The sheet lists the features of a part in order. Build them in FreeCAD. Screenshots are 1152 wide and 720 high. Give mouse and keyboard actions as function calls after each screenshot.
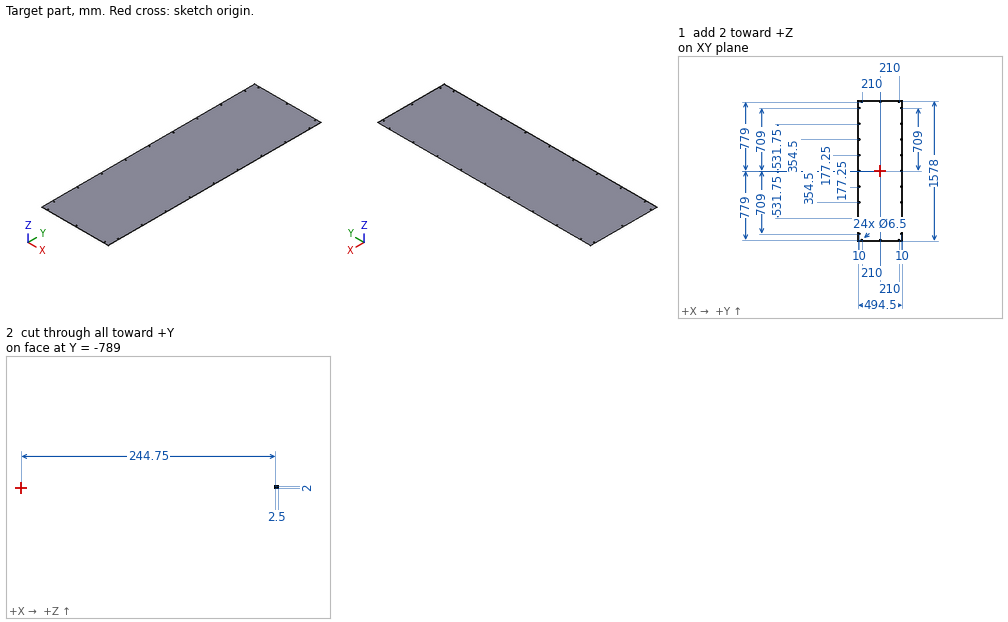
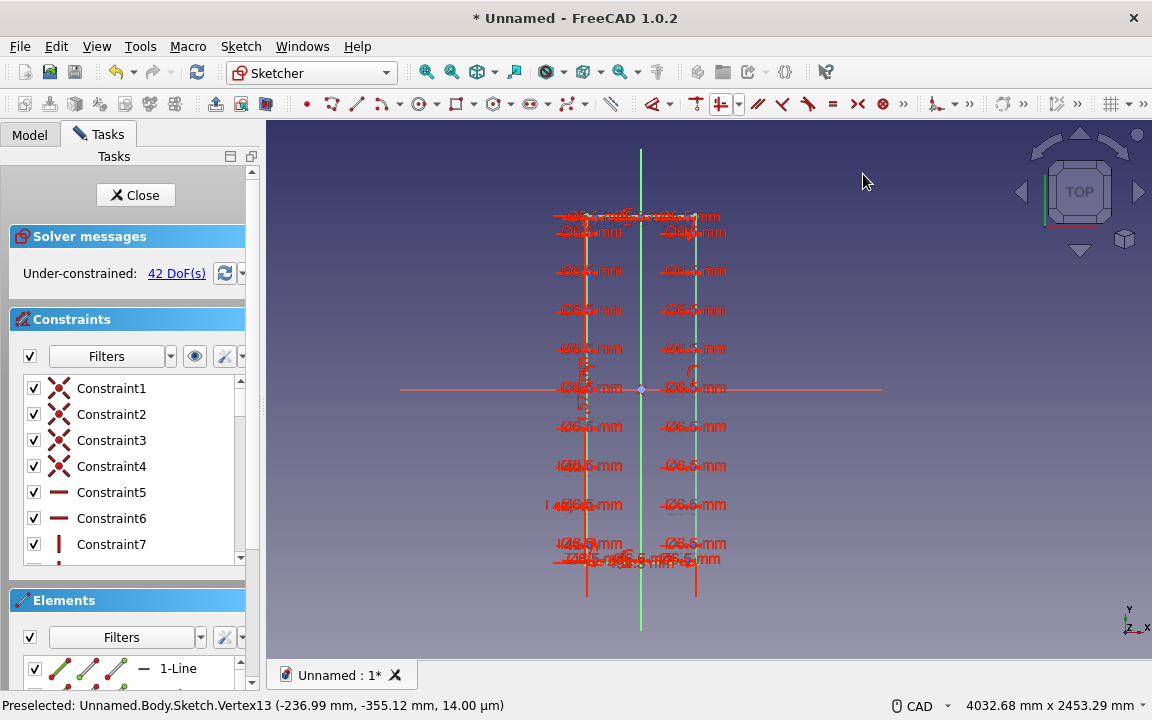
click(589, 468)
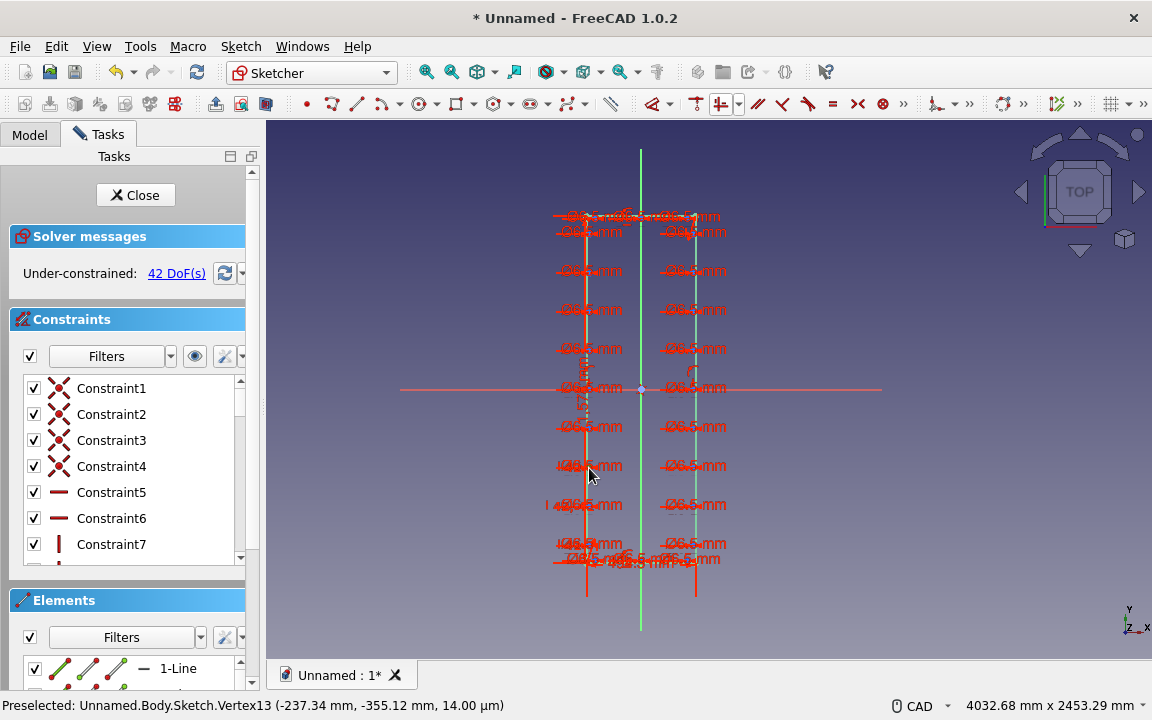
click(589, 429)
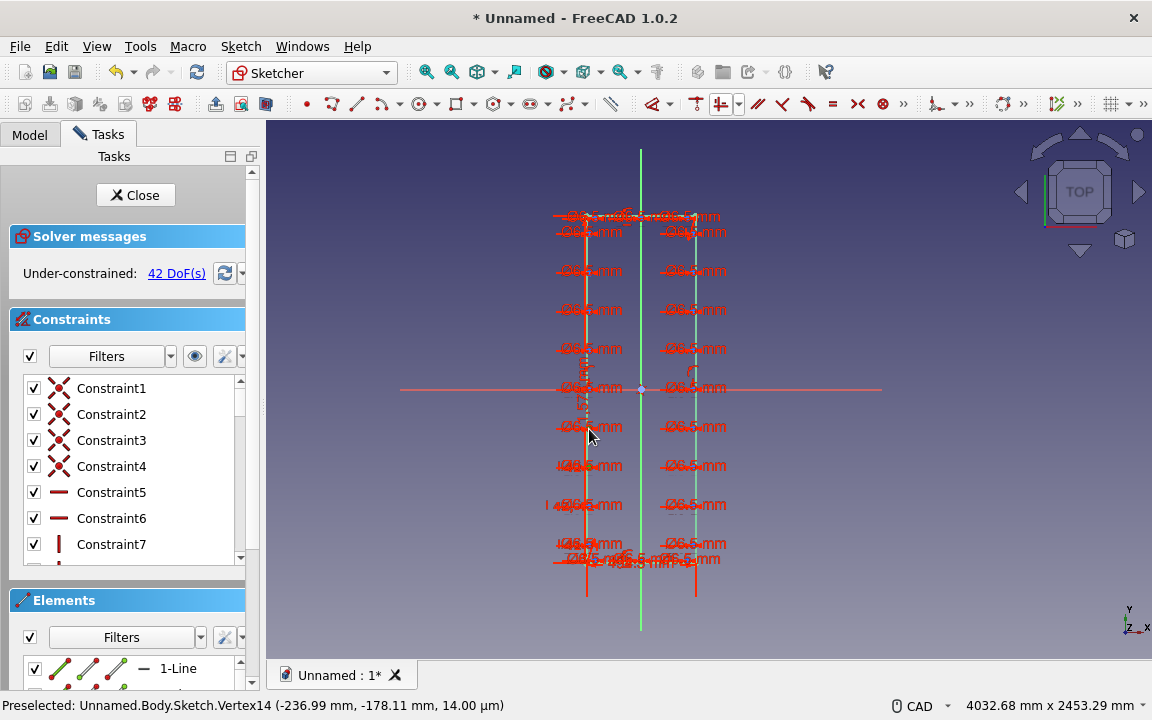
key(v)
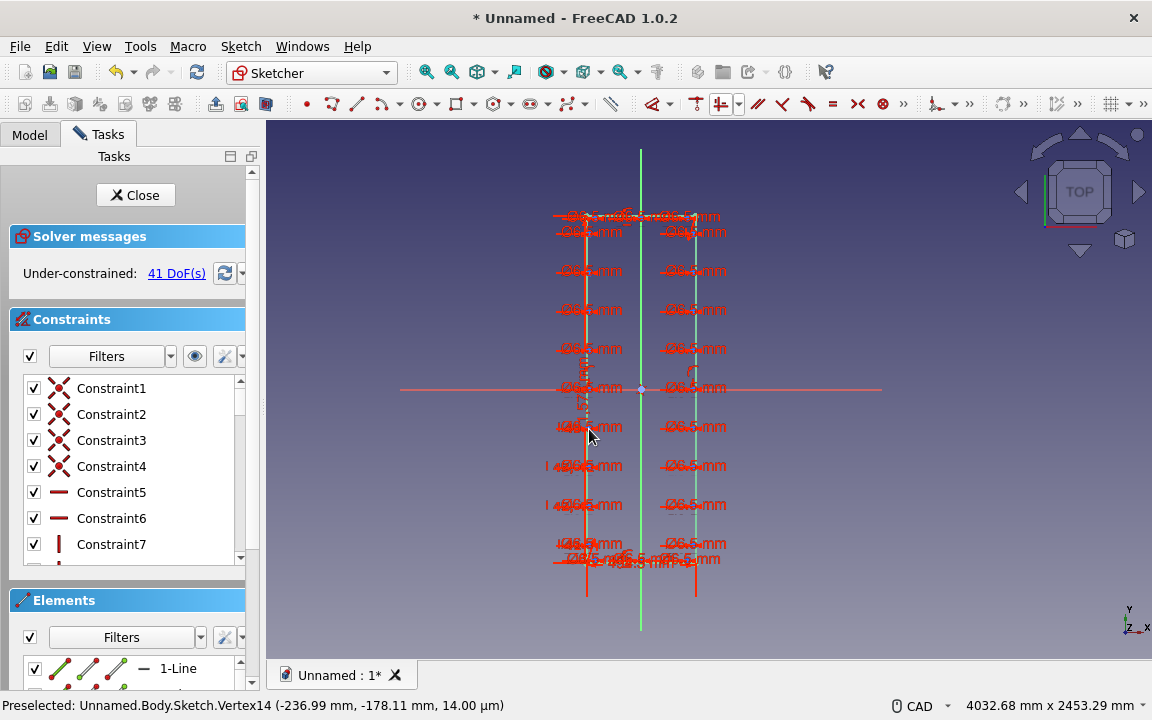
scroll(595, 561, up, 2)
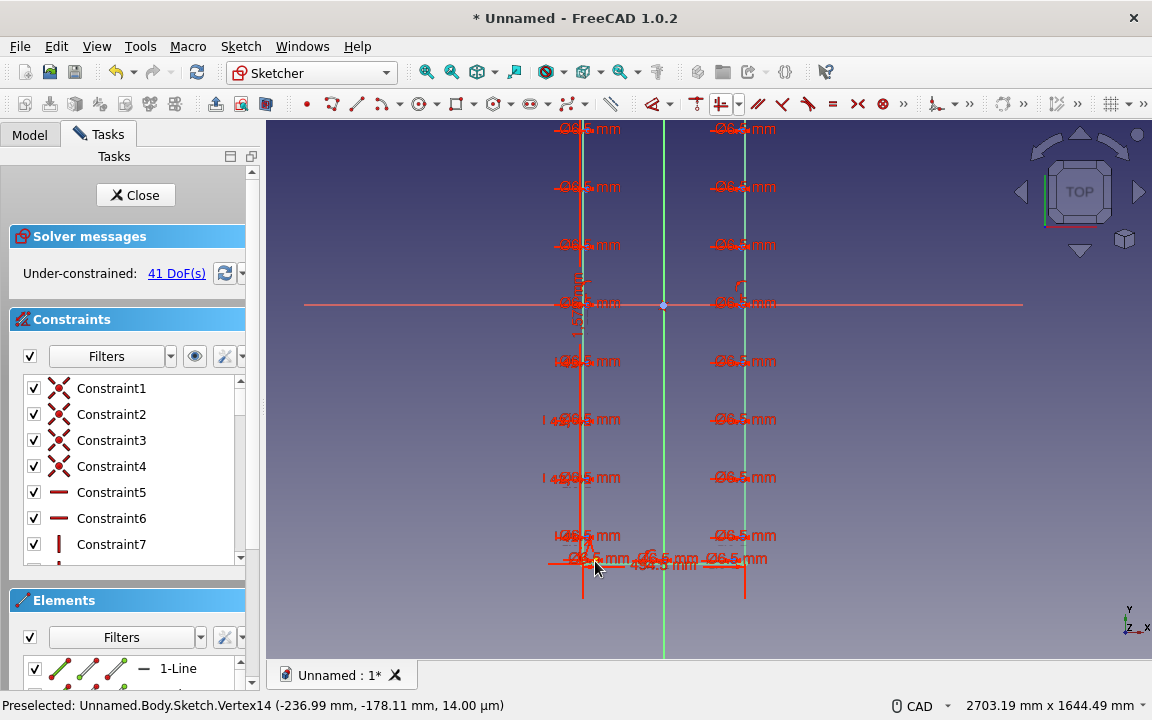
click(595, 560)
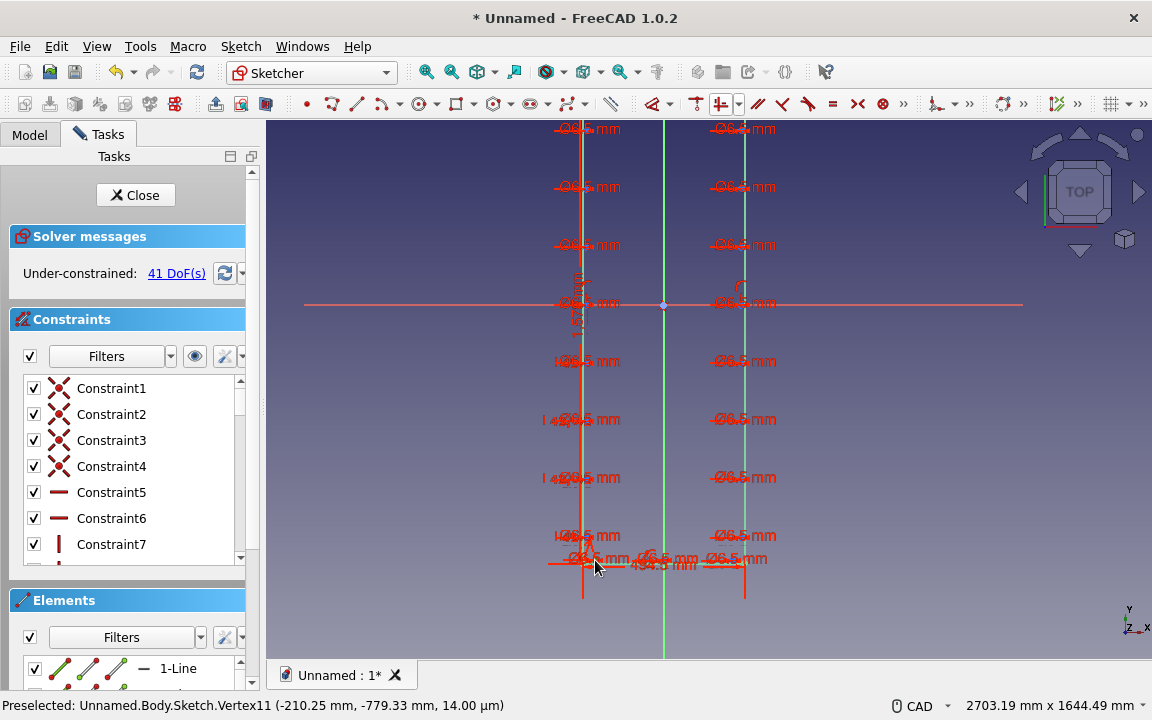
click(664, 561)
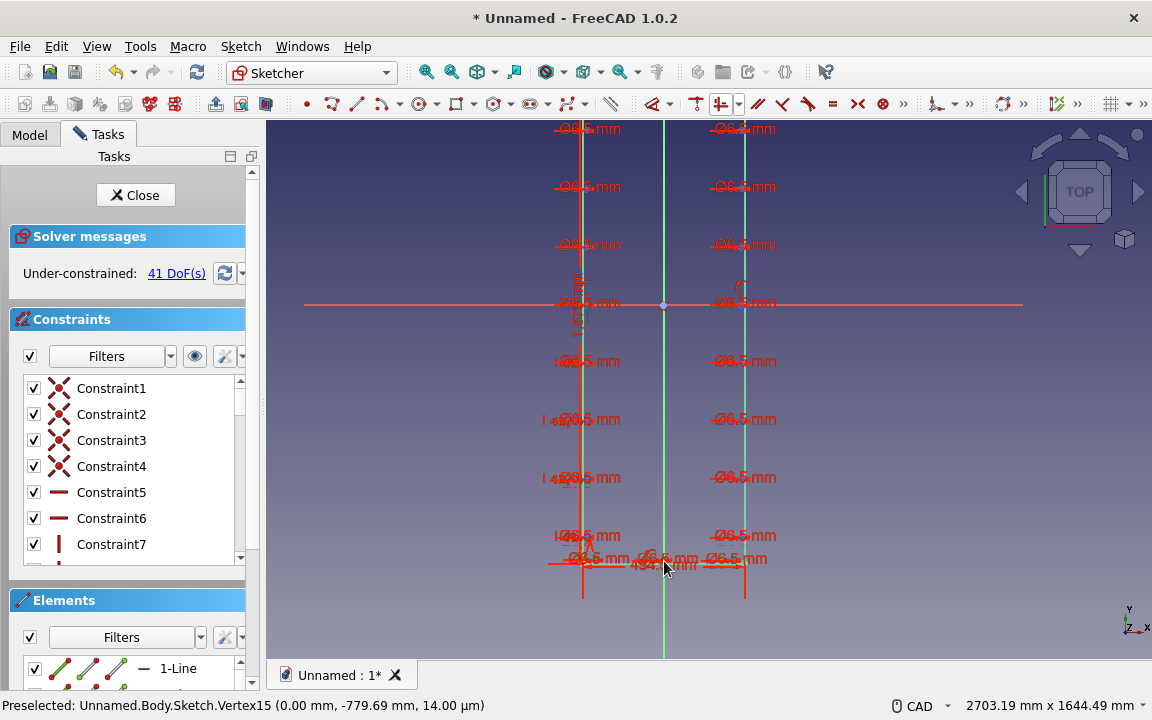
key(h)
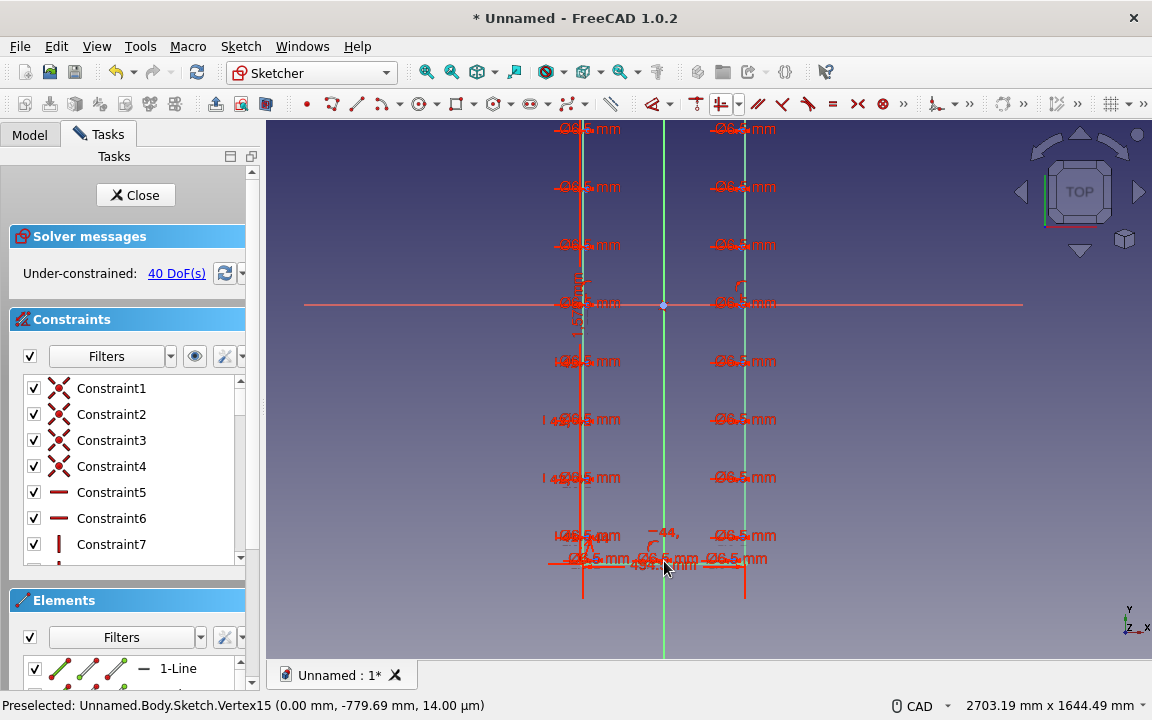
click(664, 561)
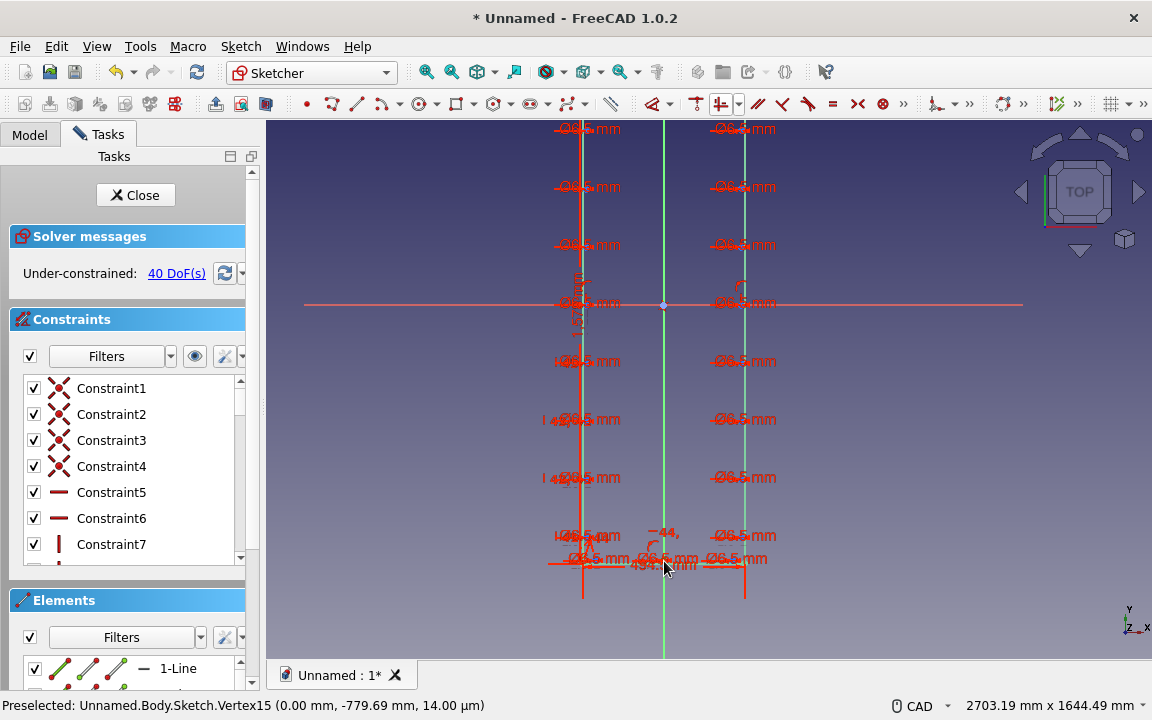
click(733, 561)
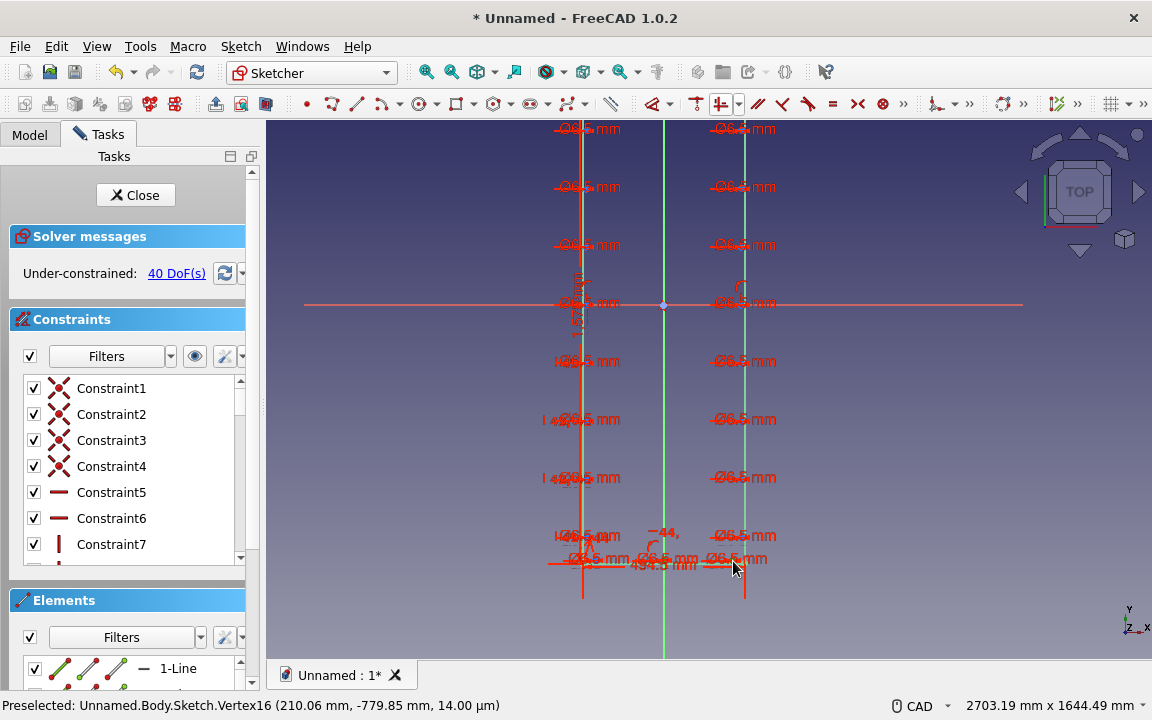
key(h)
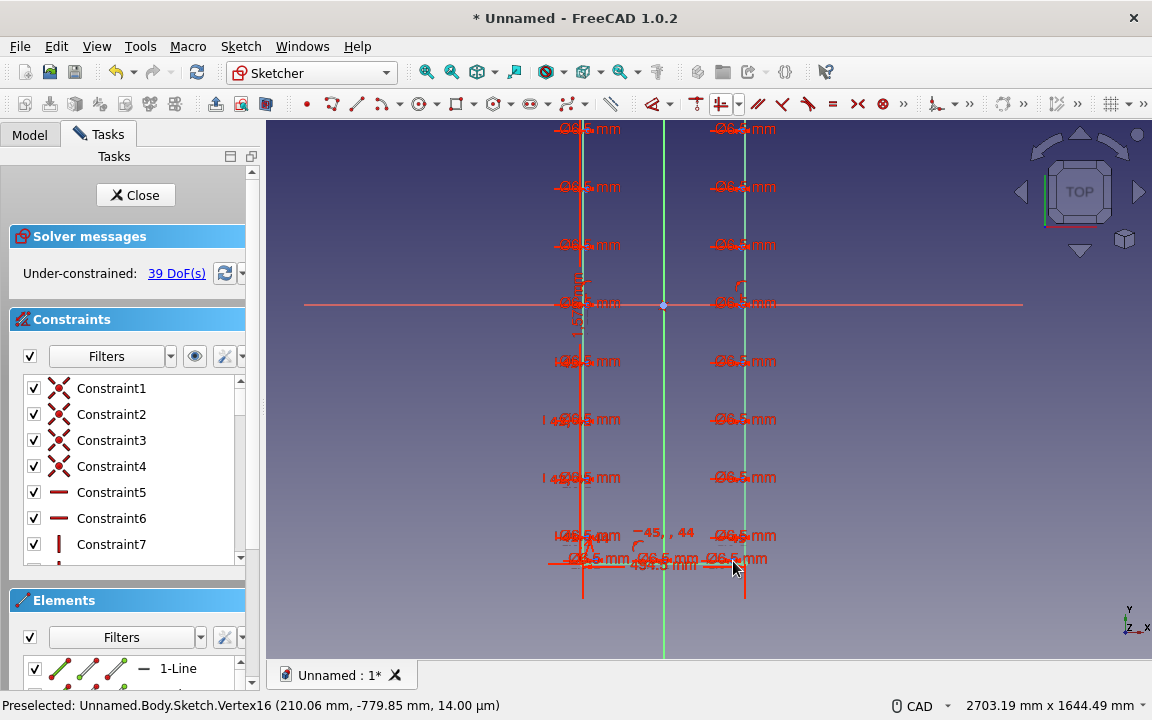
click(586, 538)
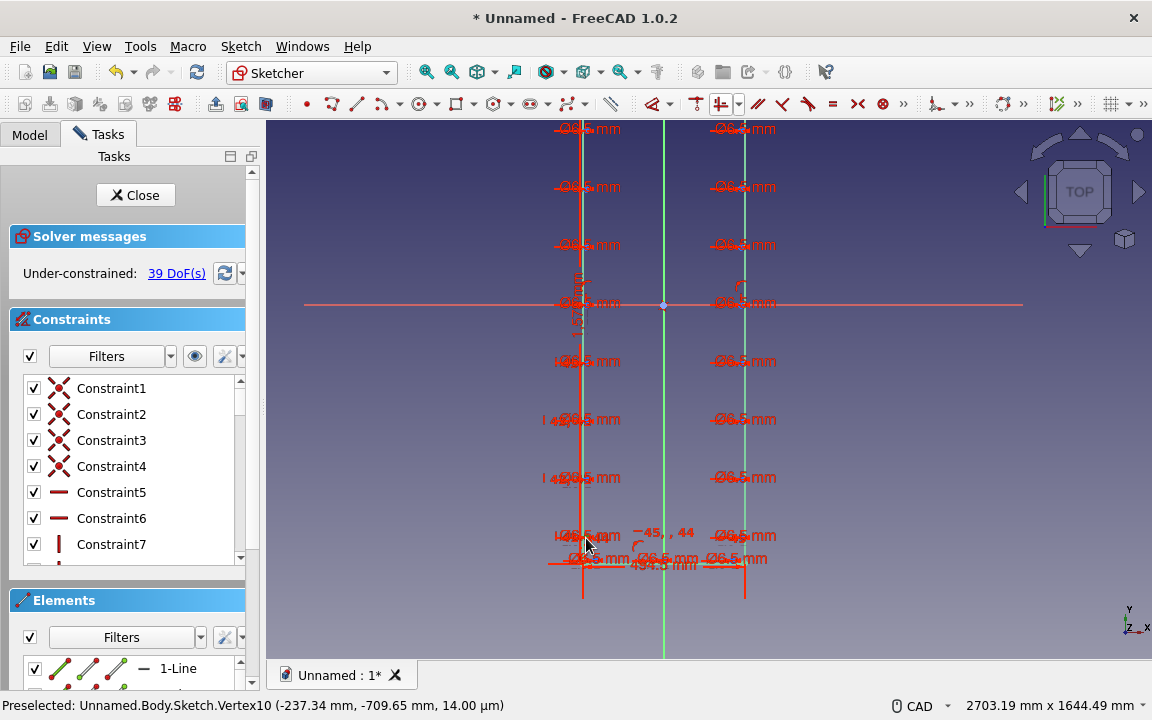
scroll(742, 538, up, 4)